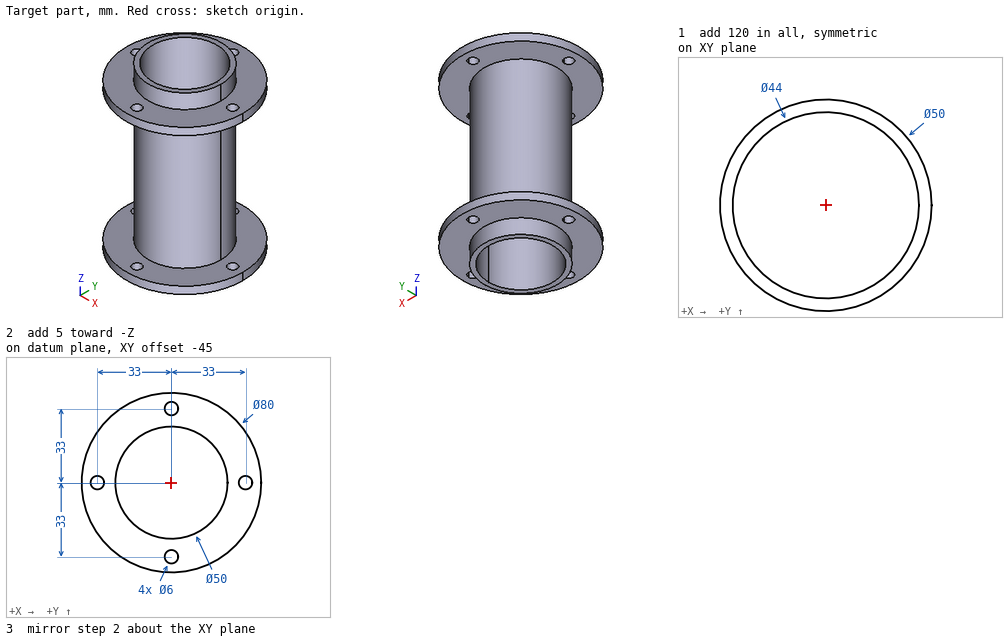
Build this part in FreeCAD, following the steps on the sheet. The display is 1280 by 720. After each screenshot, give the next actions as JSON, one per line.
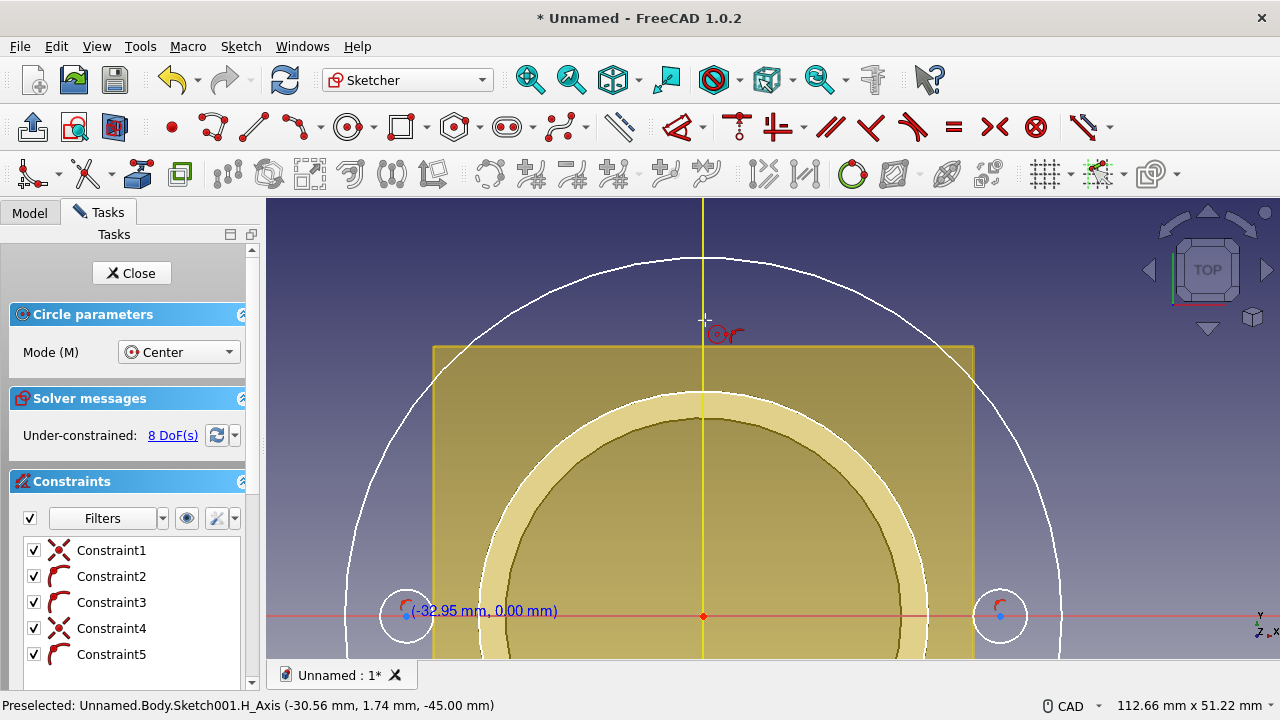
{"action": "left_click", "coordinate": [703, 319]}
{"action": "left_click", "coordinate": [722, 300]}
{"action": "key", "text": "Escape"}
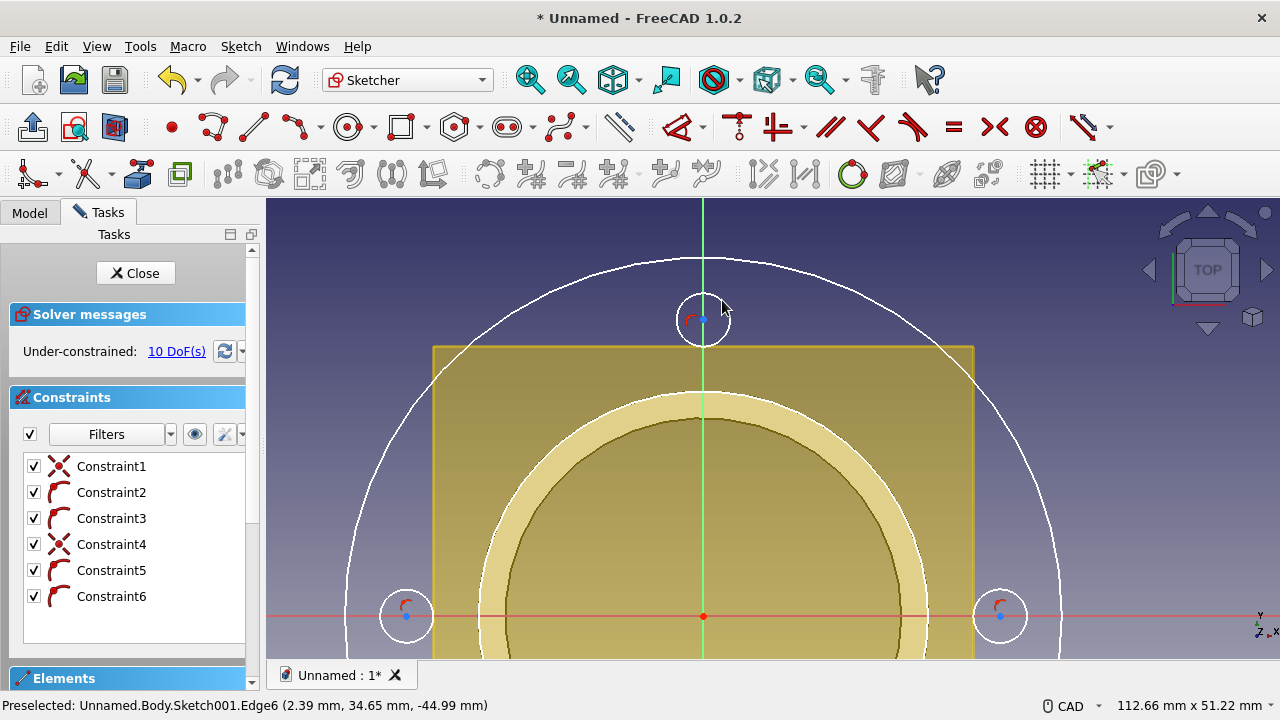
{"action": "scroll", "coordinate": [705, 319], "scroll_direction": "down", "scroll_amount": 5}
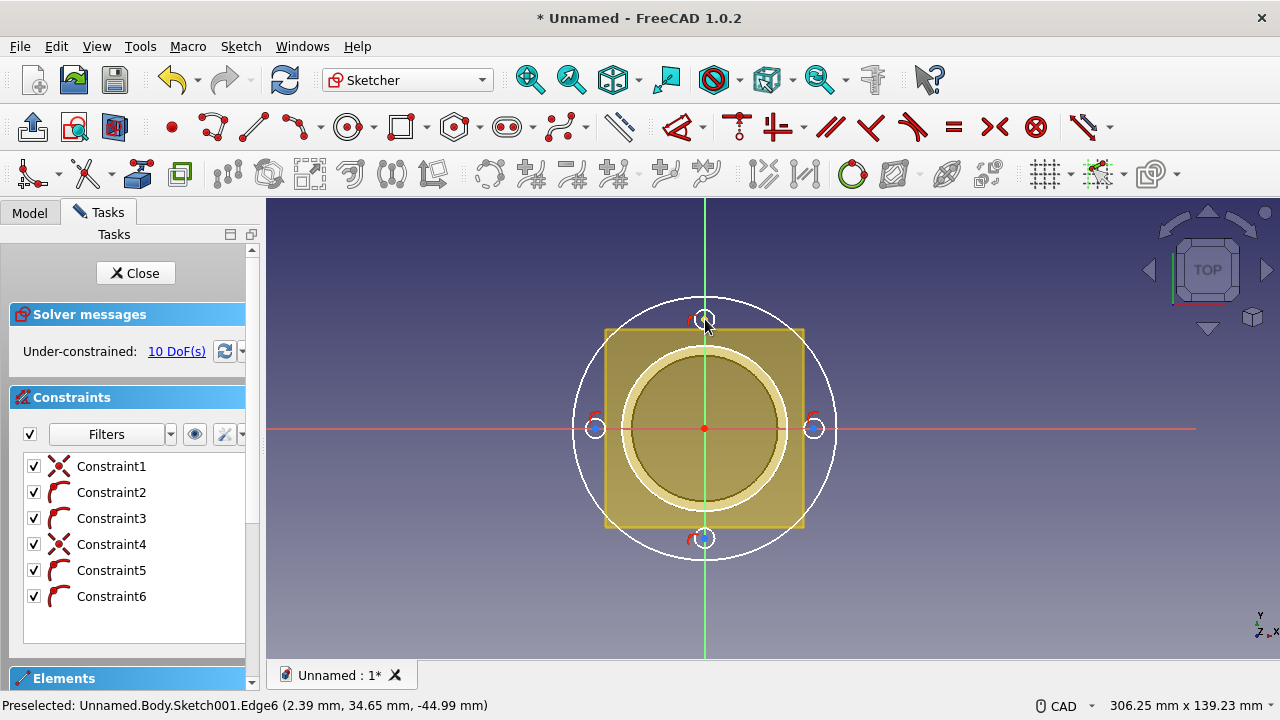
{"action": "scroll", "coordinate": [712, 531], "scroll_direction": "up", "scroll_amount": 4}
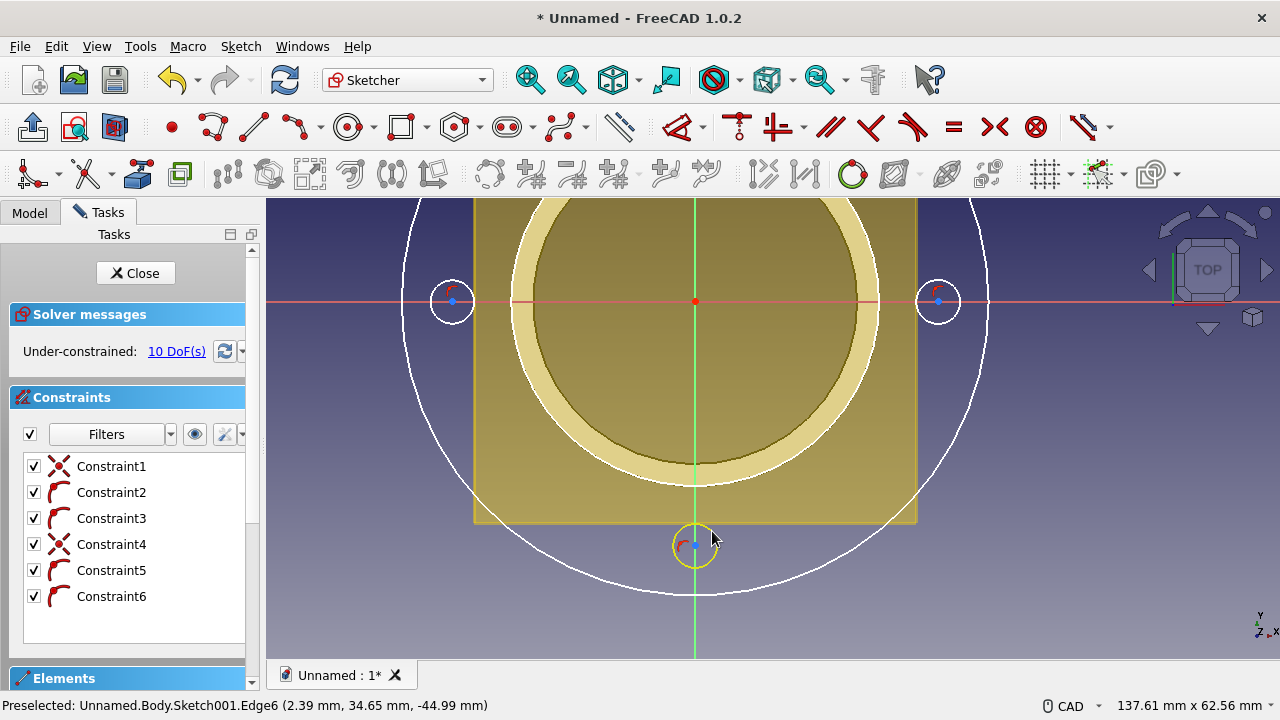
{"action": "left_click", "coordinate": [711, 530]}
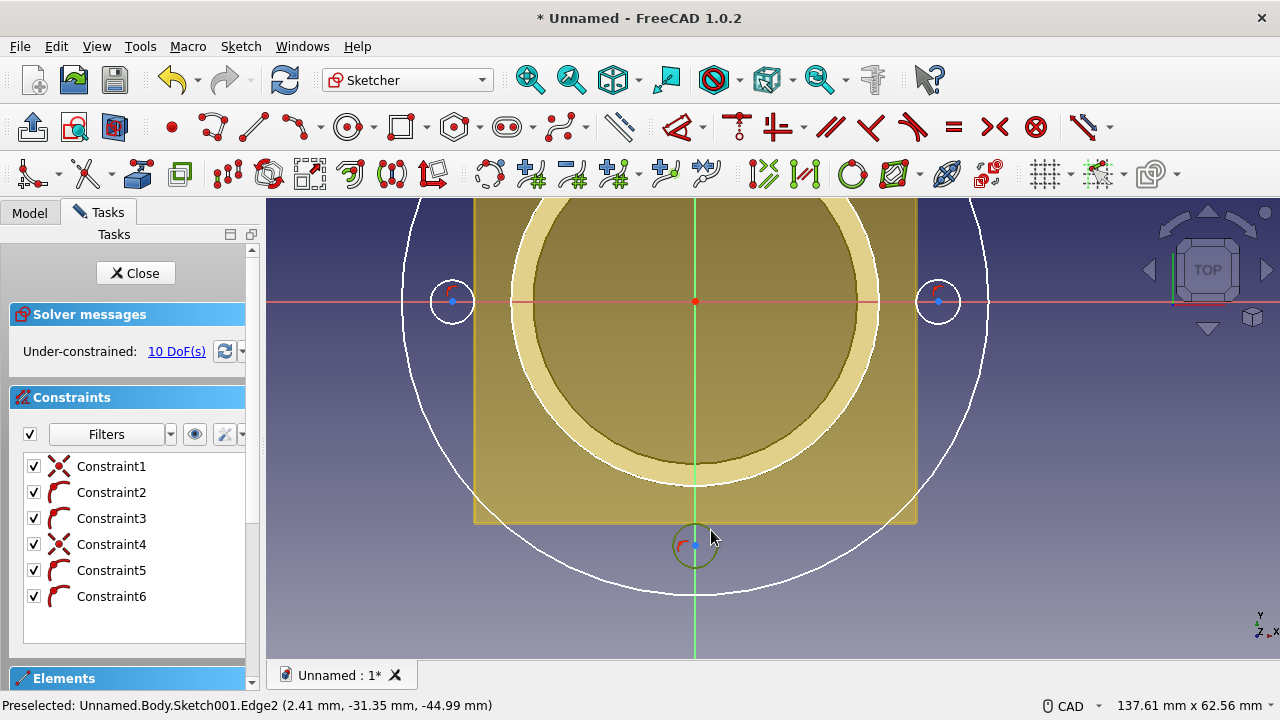
{"action": "left_click", "coordinate": [954, 286]}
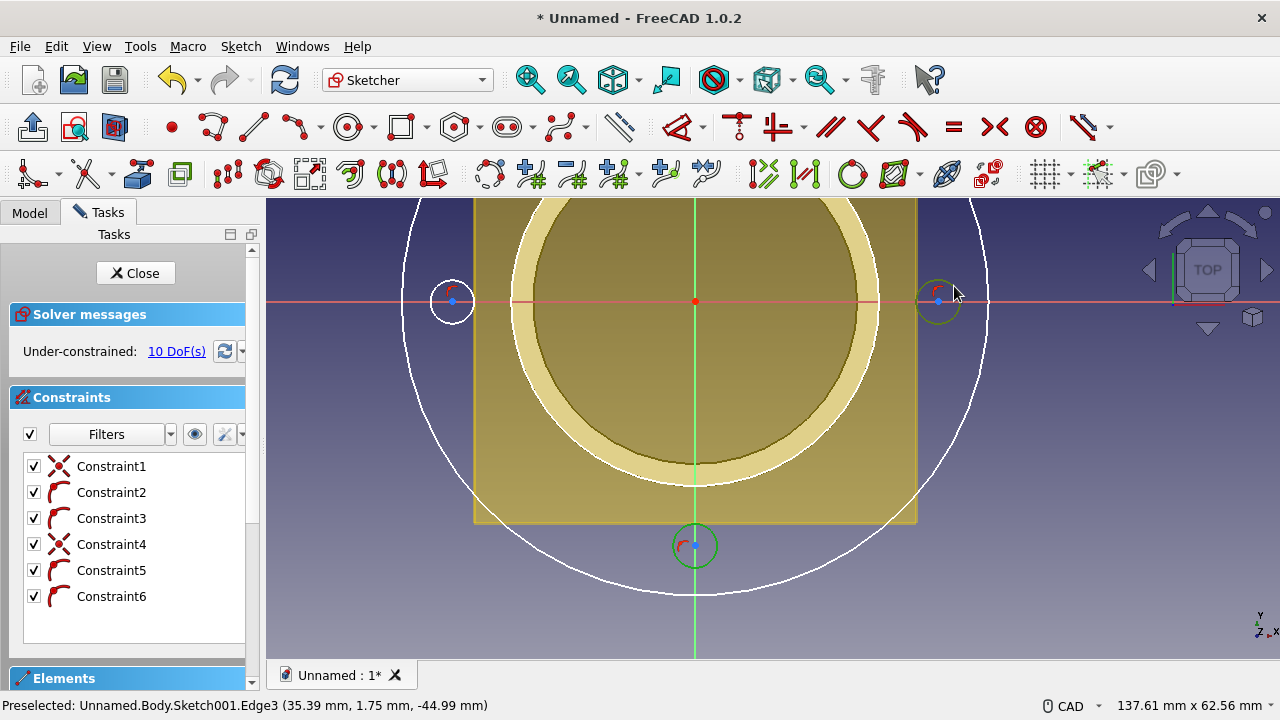
{"action": "left_click", "coordinate": [468, 287]}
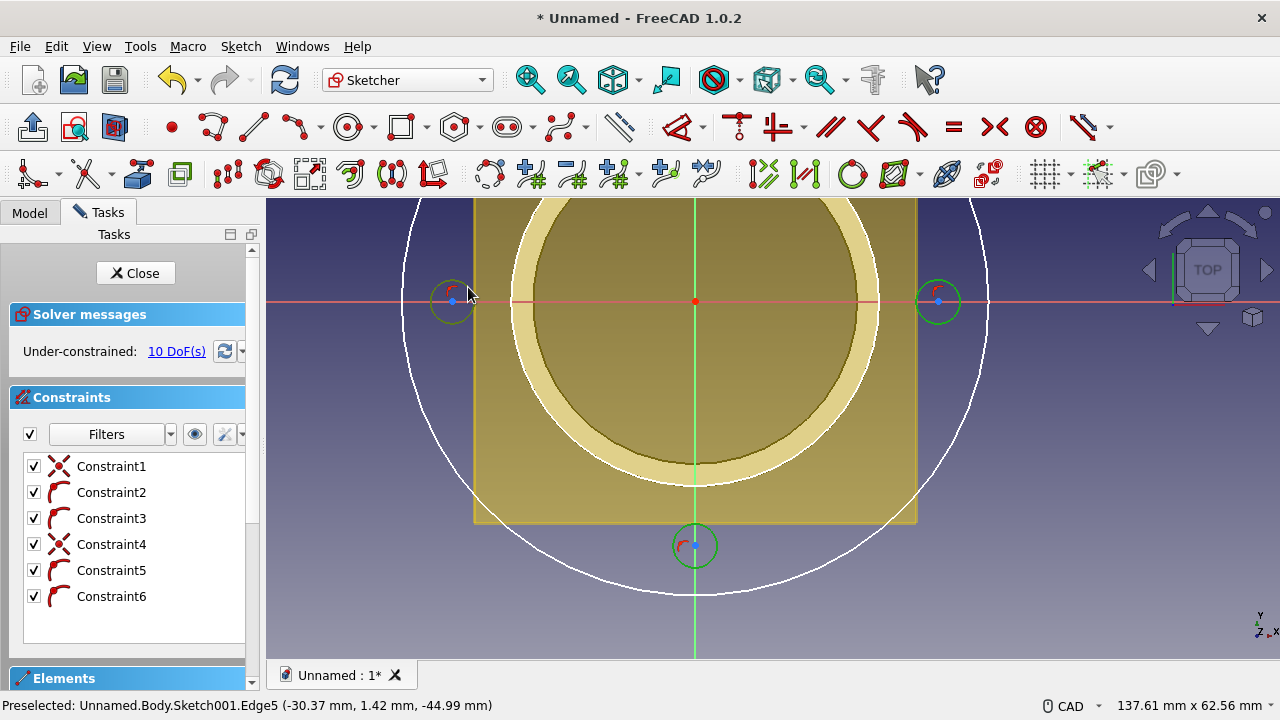
{"action": "scroll", "coordinate": [712, 532], "scroll_direction": "down", "scroll_amount": 4}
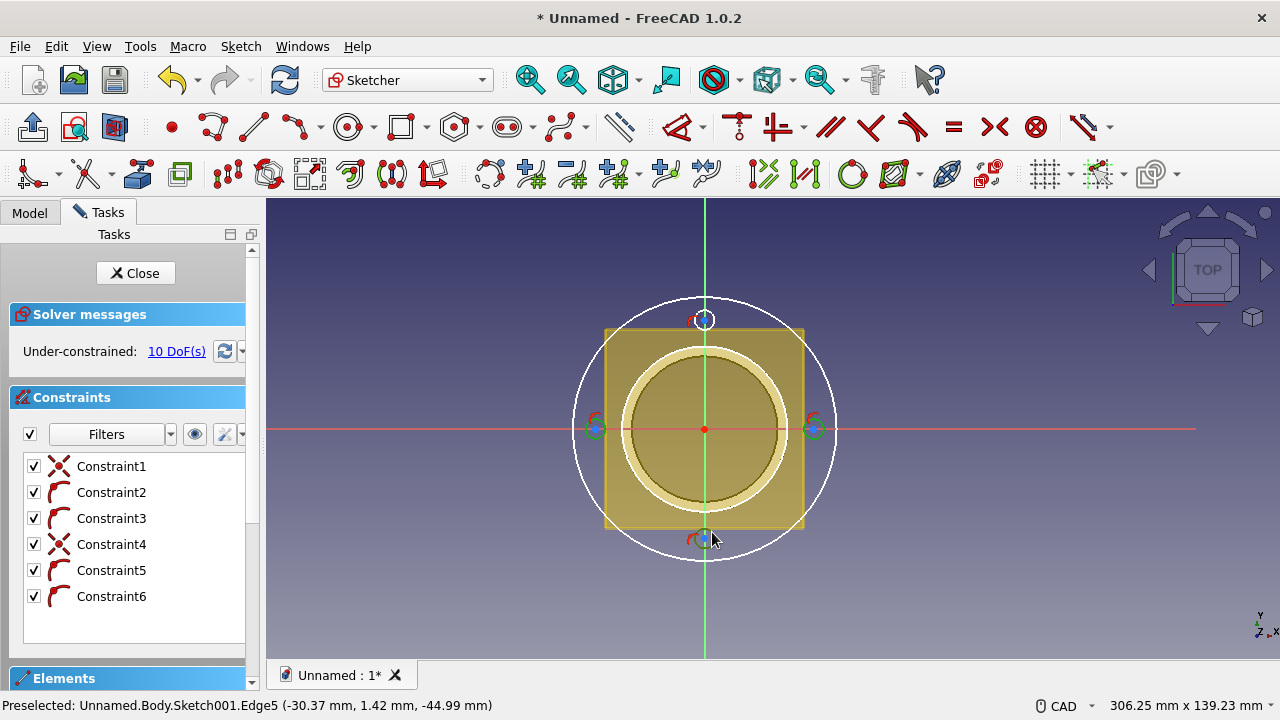
{"action": "scroll", "coordinate": [712, 313], "scroll_direction": "up", "scroll_amount": 4}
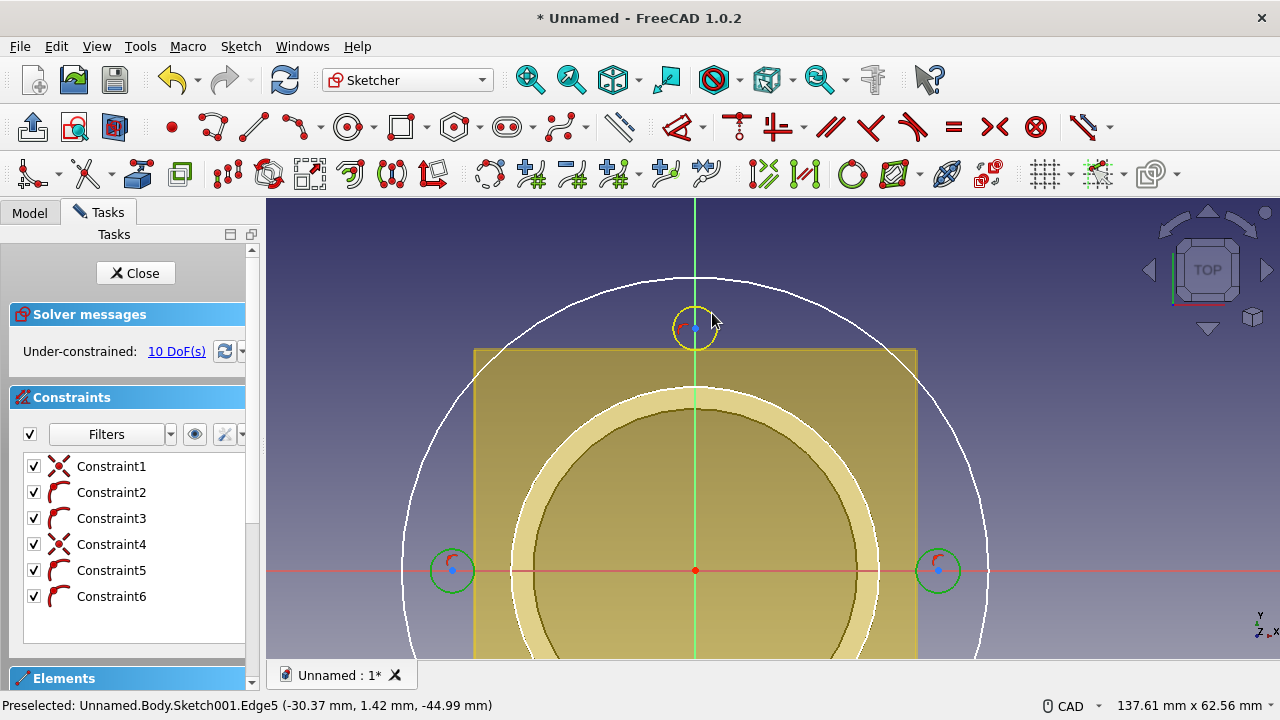
{"action": "left_click", "coordinate": [711, 313]}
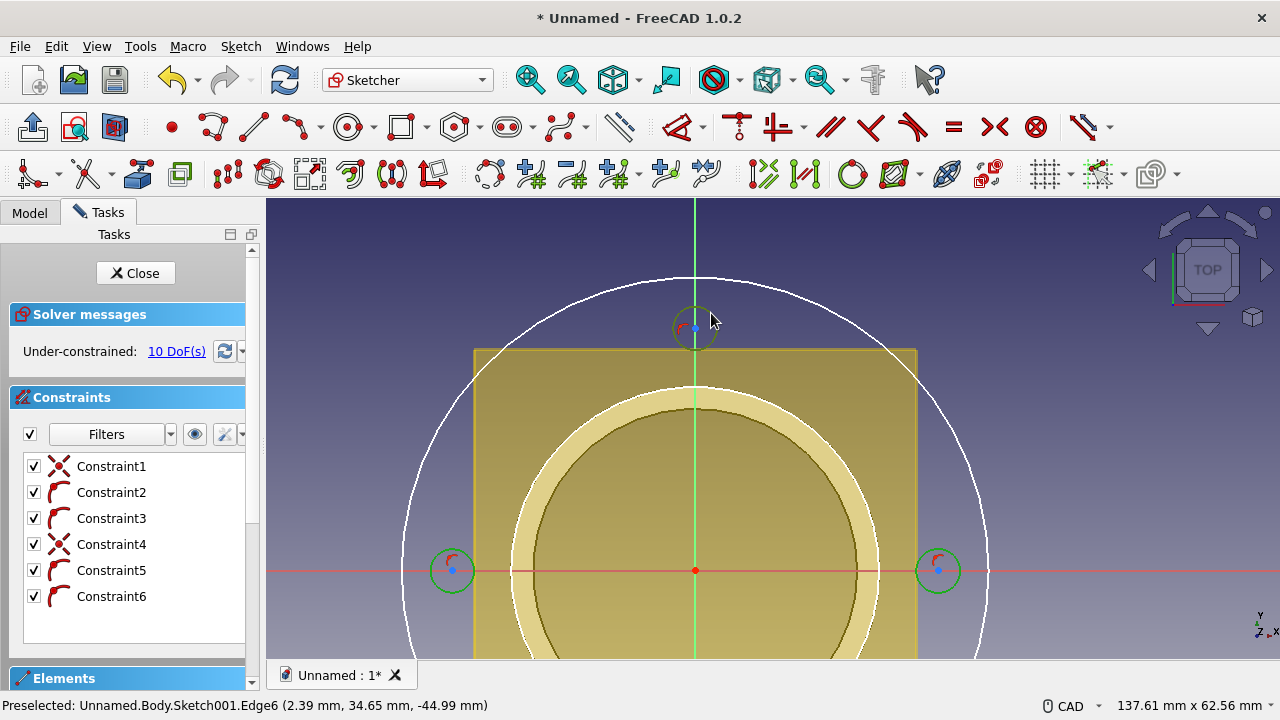
{"action": "left_click", "coordinate": [954, 128]}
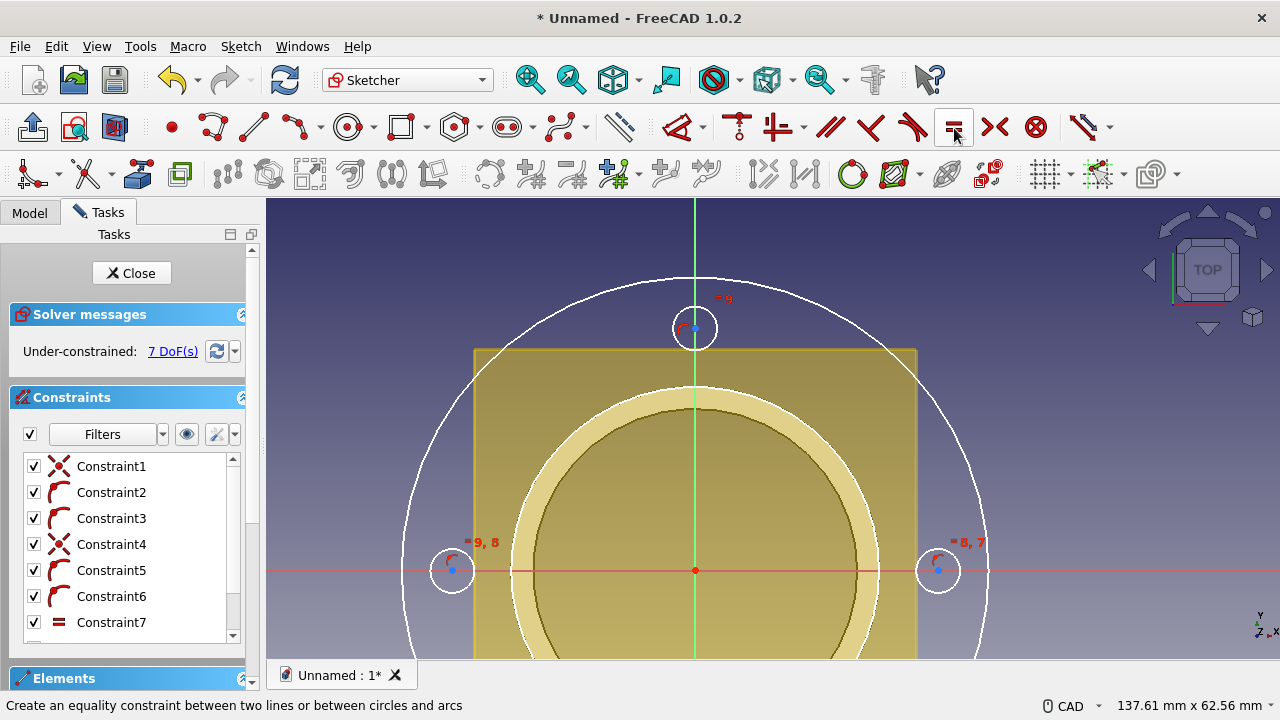
{"action": "left_click", "coordinate": [676, 128]}